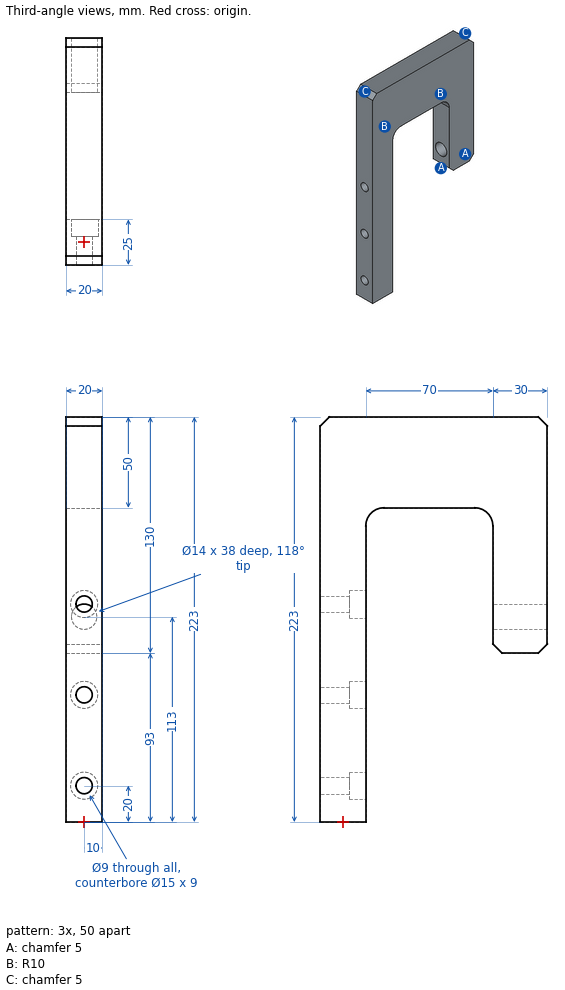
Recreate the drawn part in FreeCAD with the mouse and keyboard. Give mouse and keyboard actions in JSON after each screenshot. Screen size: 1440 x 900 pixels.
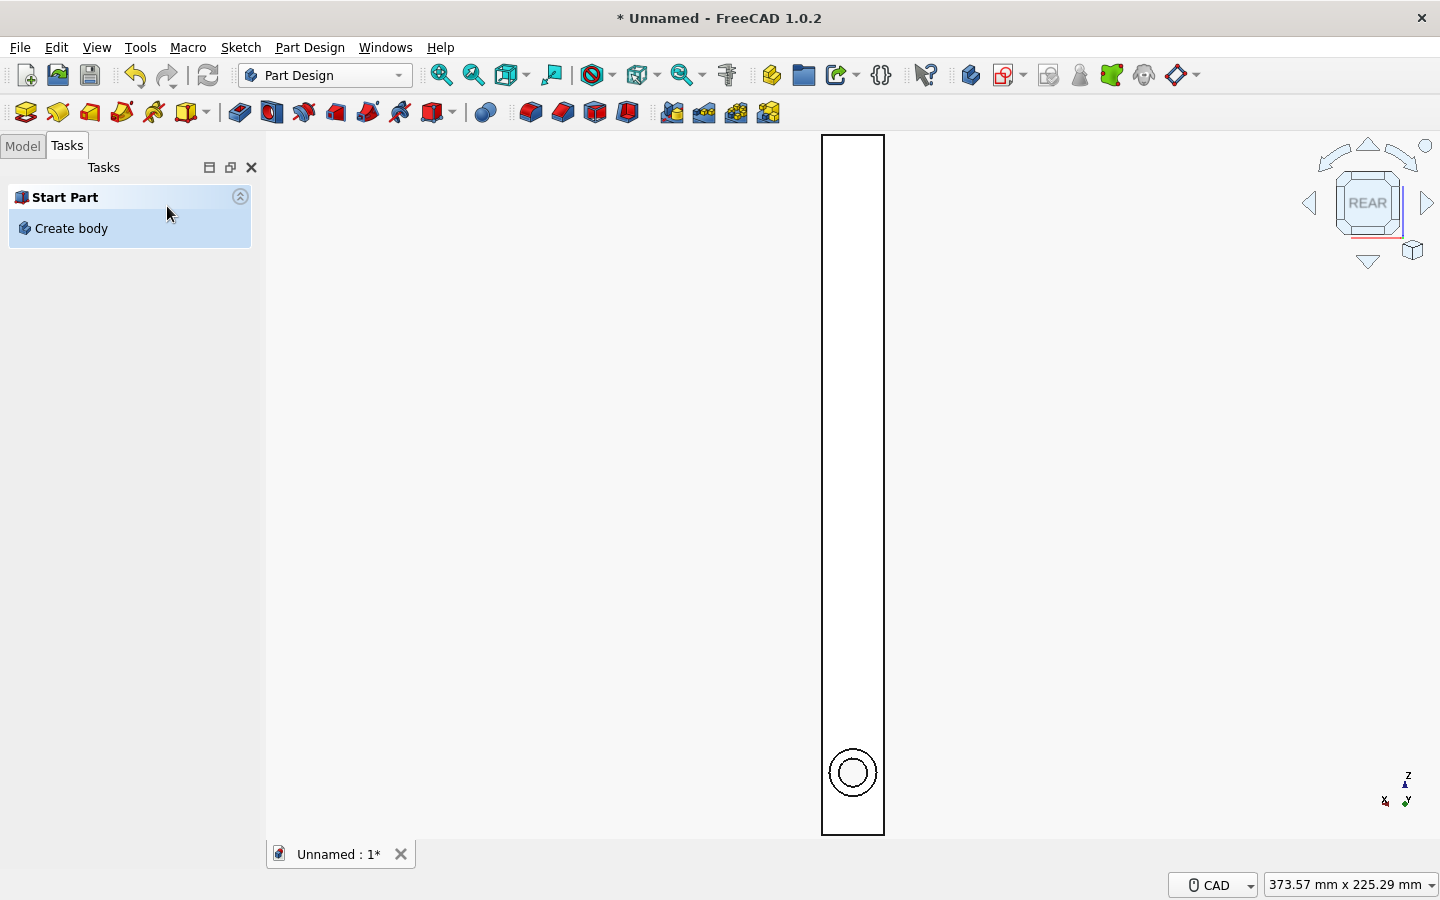
{"action": "left_click", "coordinate": [23, 145]}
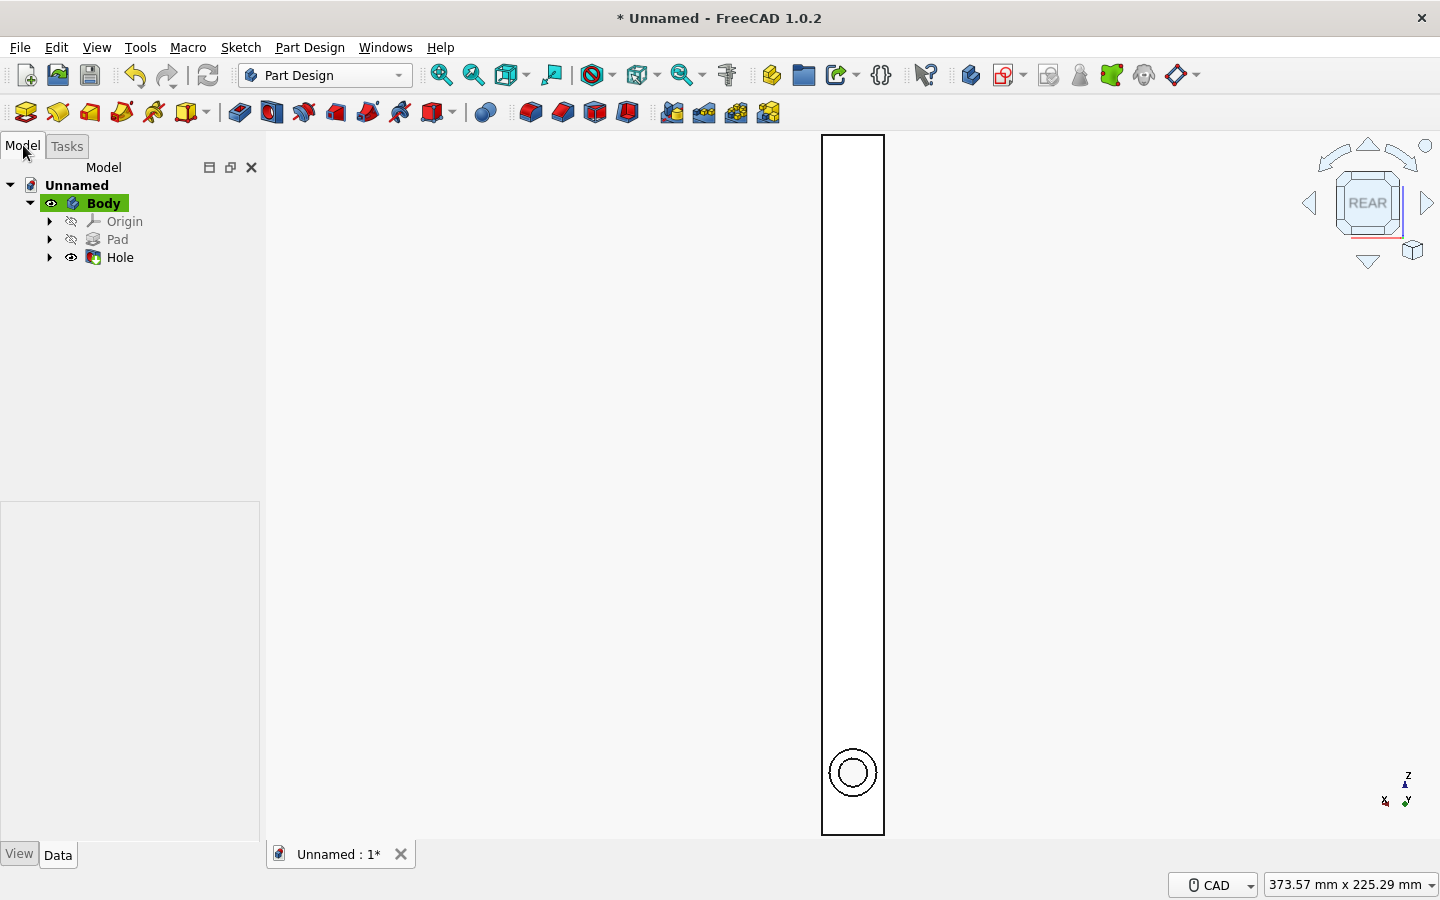
{"action": "left_click", "coordinate": [116, 257]}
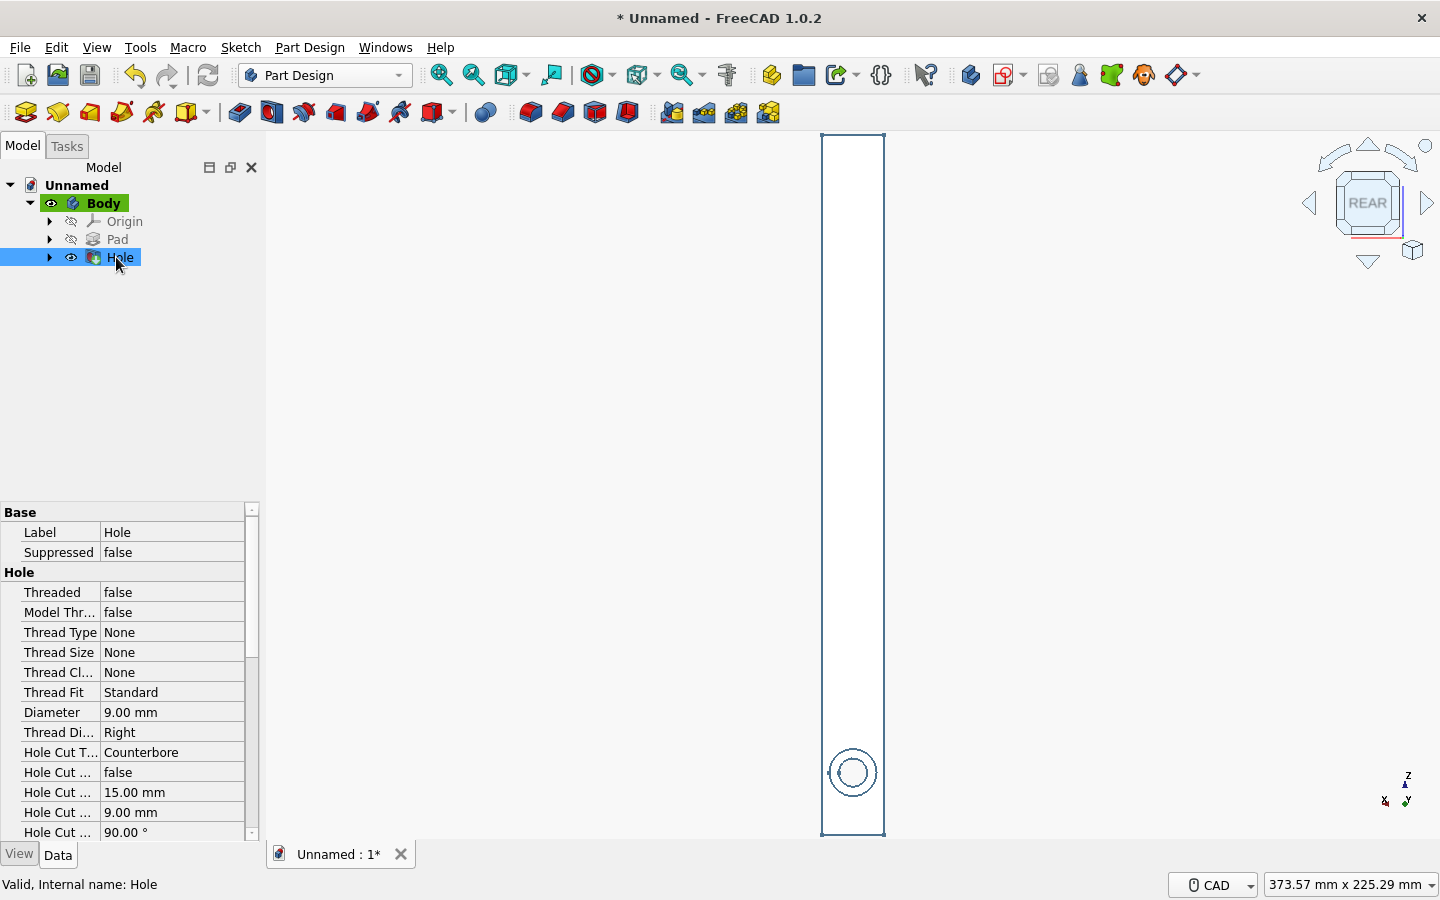
{"action": "left_click", "coordinate": [704, 112]}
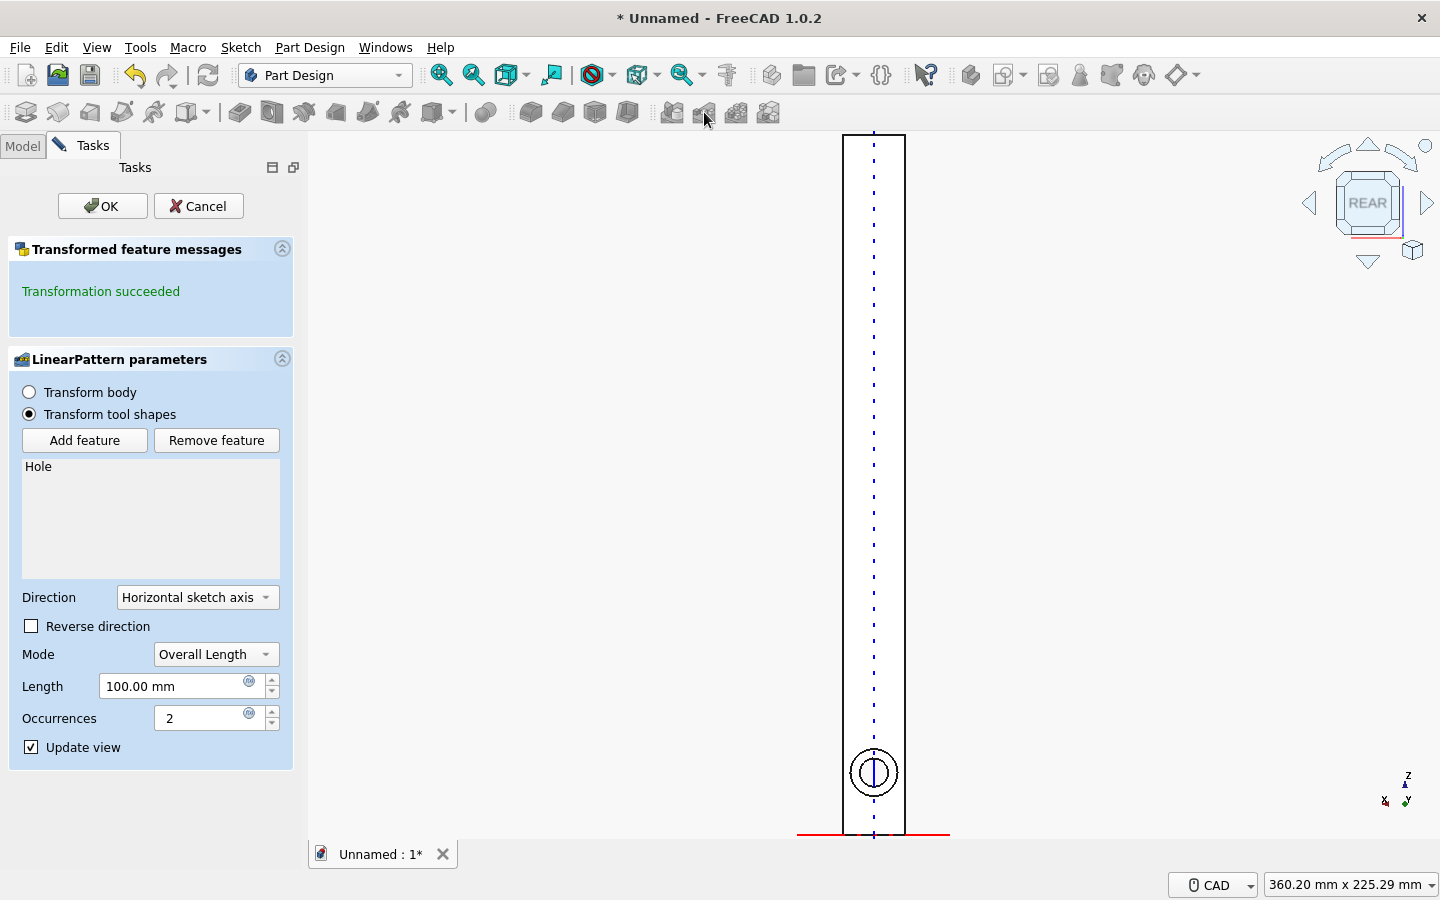
{"action": "left_click", "coordinate": [198, 598]}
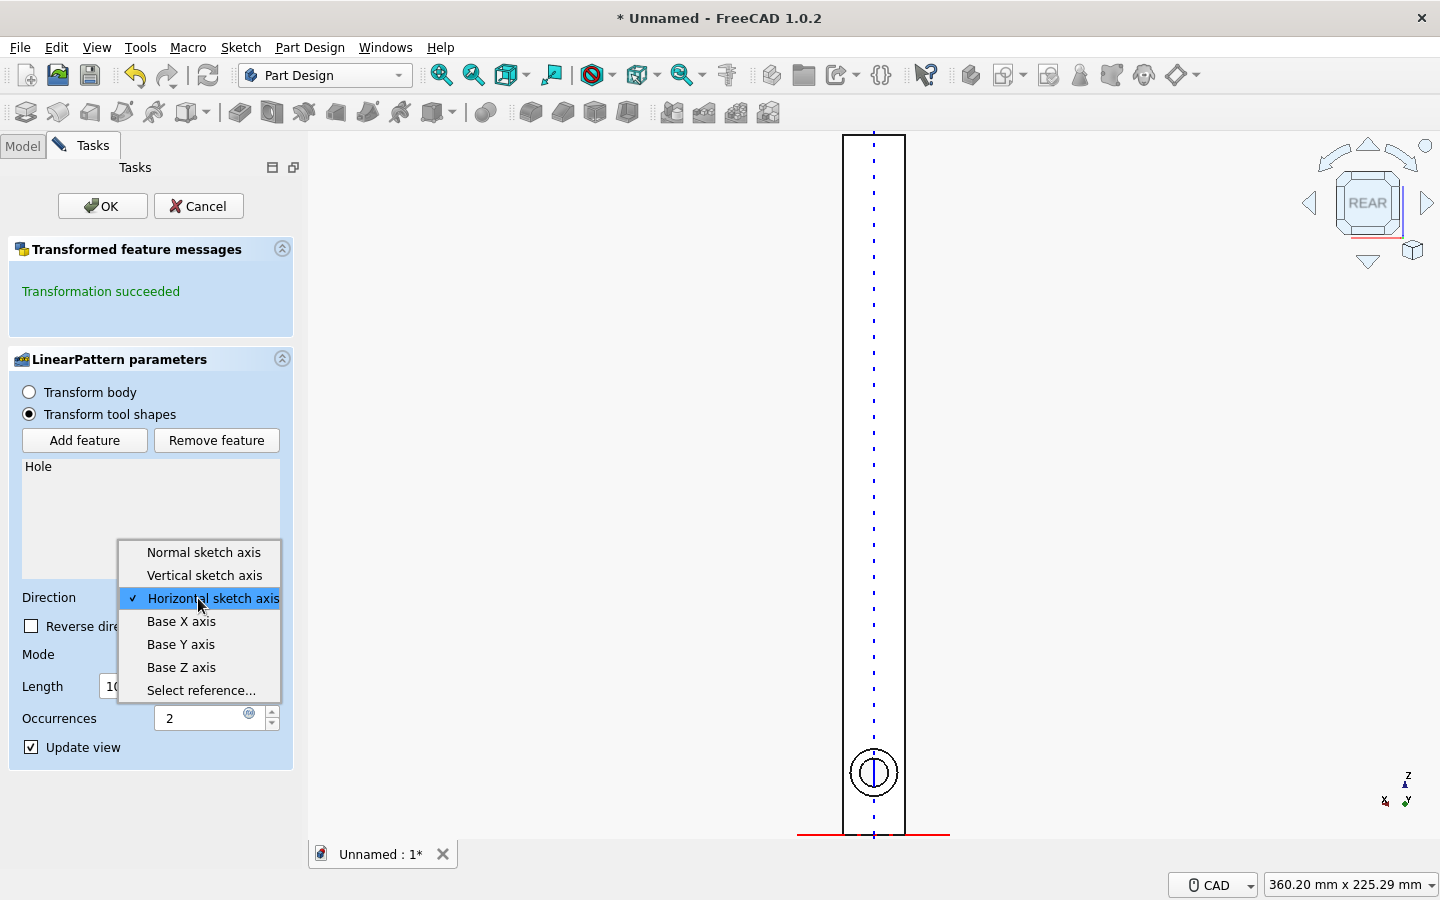
{"action": "left_click", "coordinate": [198, 668]}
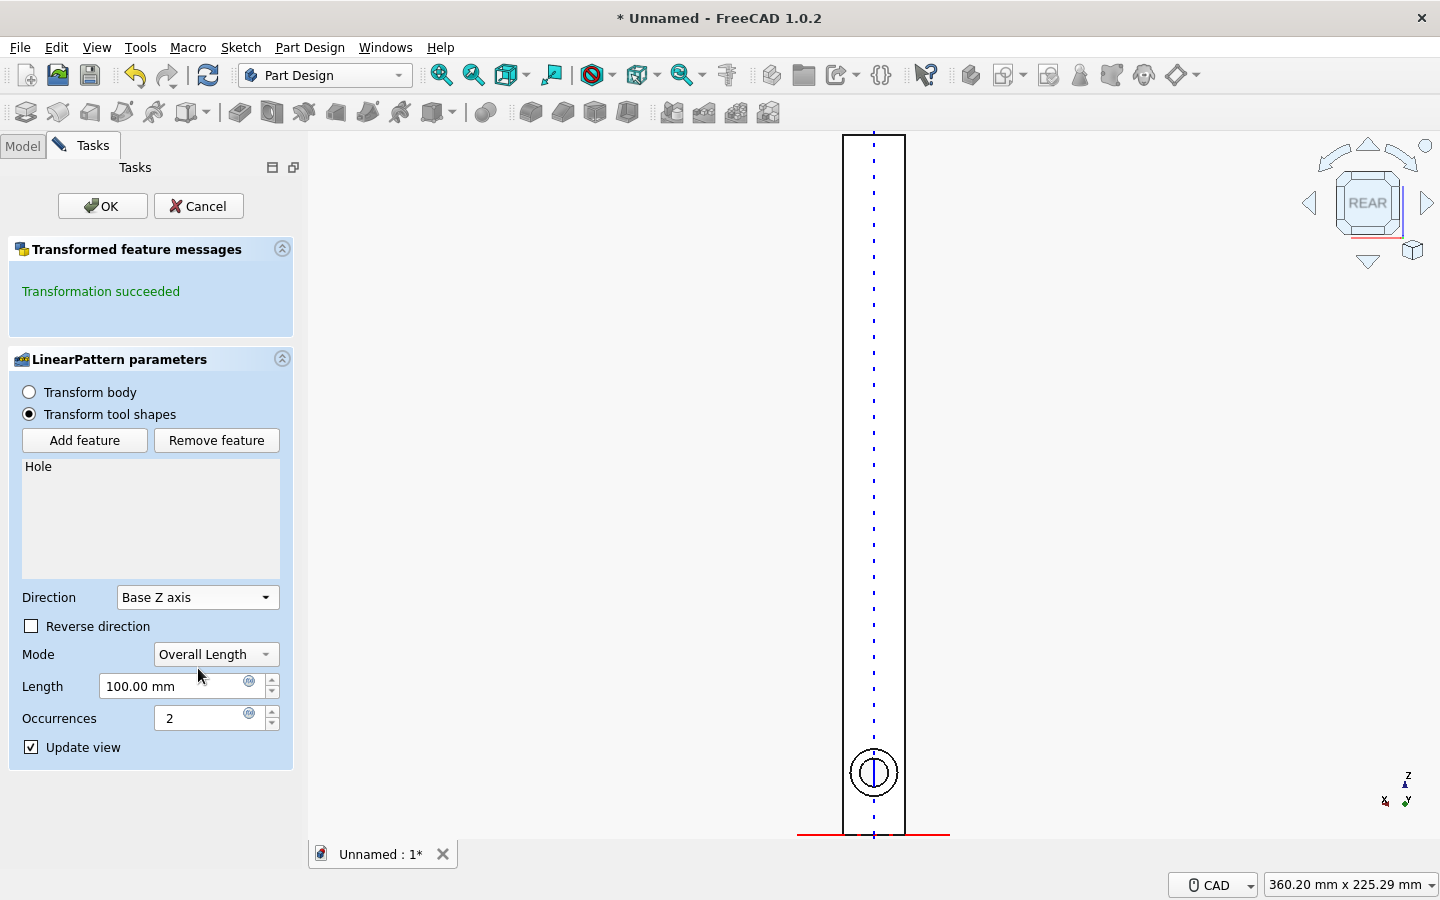
{"action": "left_click", "coordinate": [217, 654]}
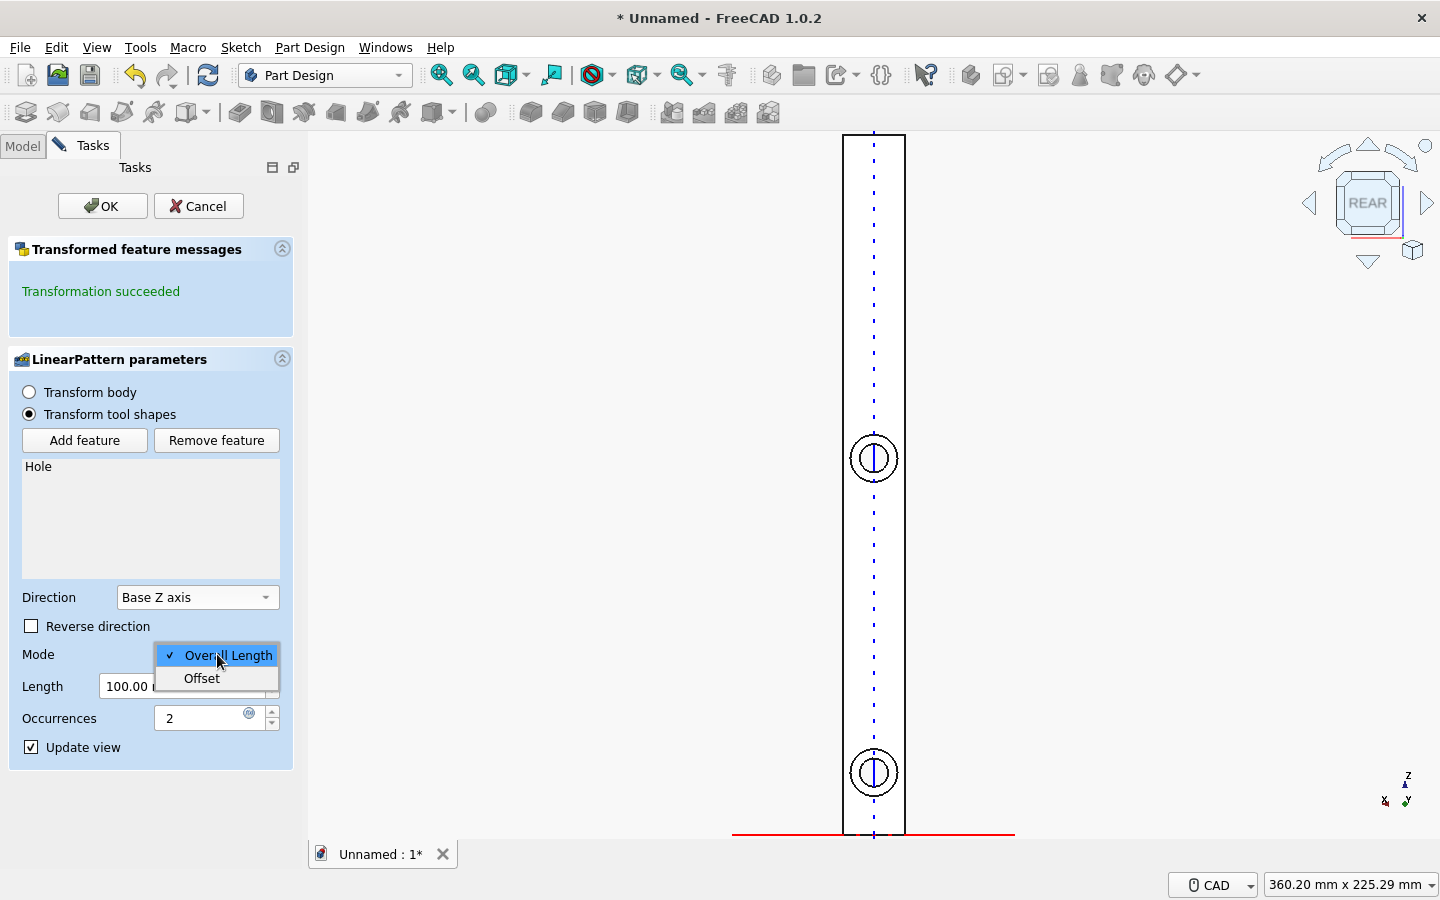
{"action": "left_click", "coordinate": [216, 678]}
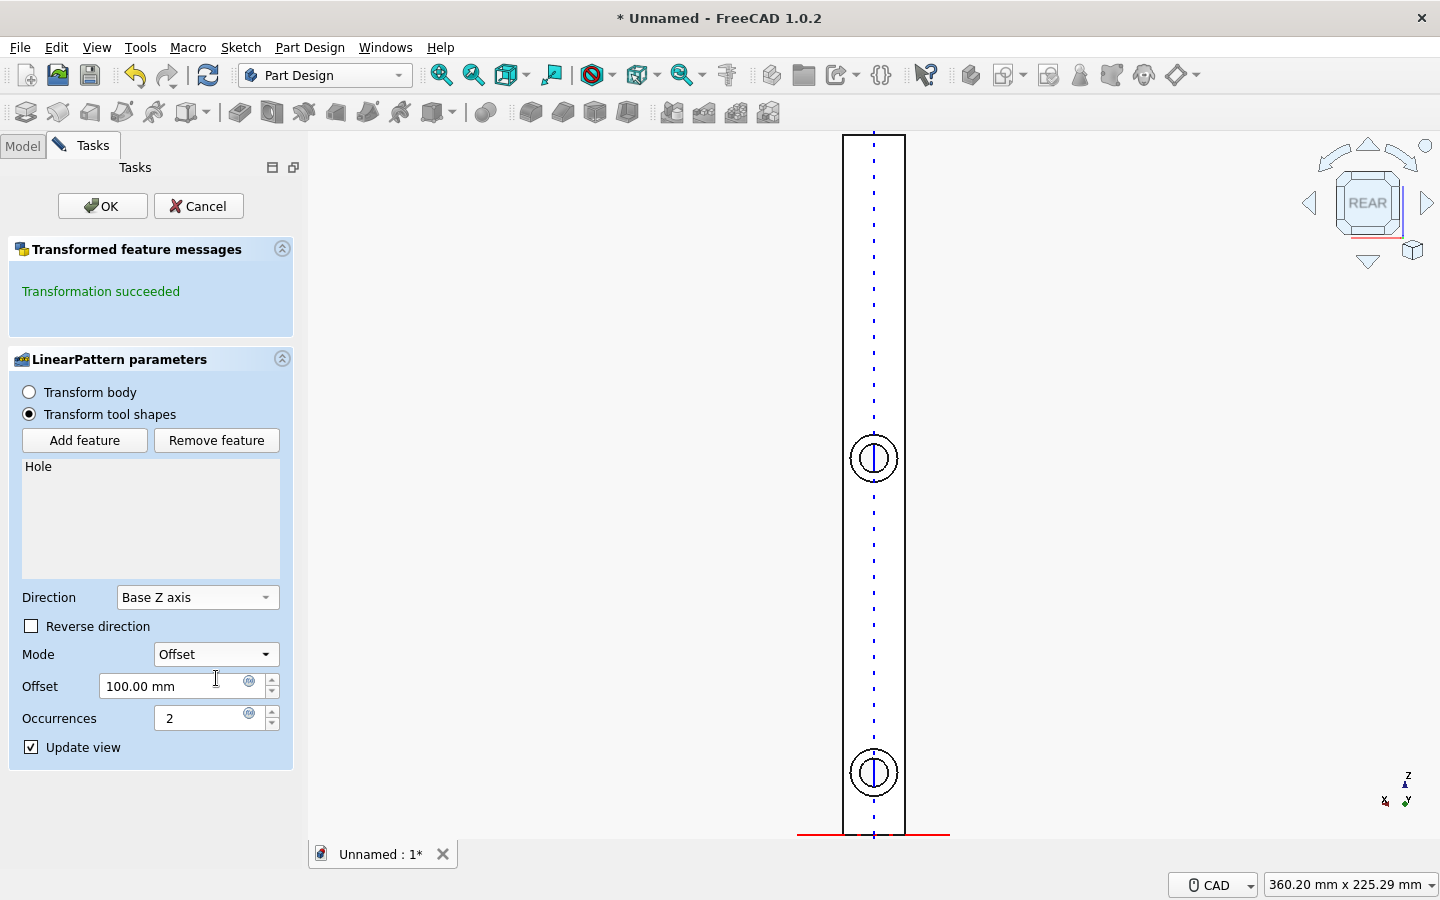
{"action": "triple_click", "coordinate": [182, 686]}